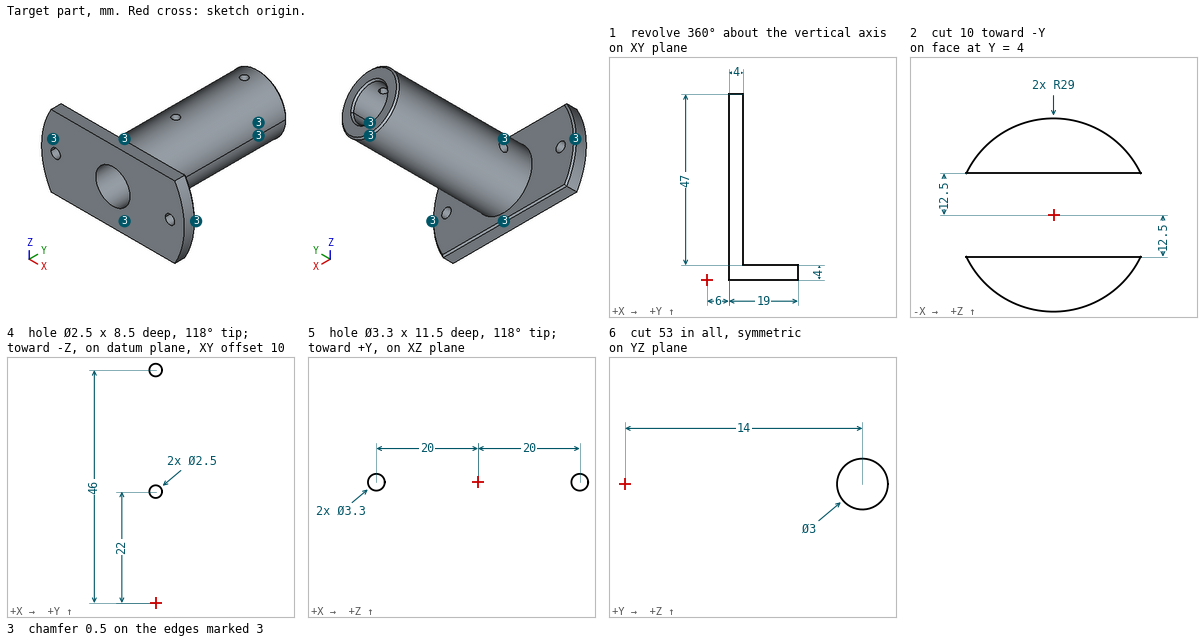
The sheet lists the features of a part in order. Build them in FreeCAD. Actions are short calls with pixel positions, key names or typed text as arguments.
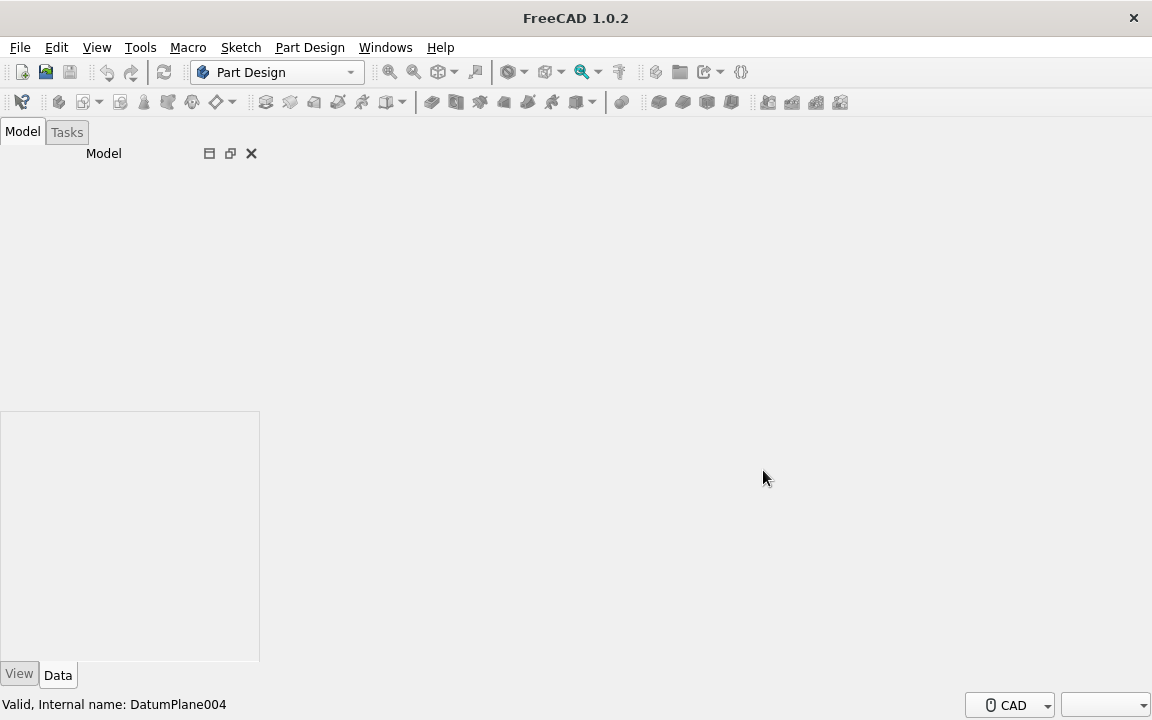
click(22, 72)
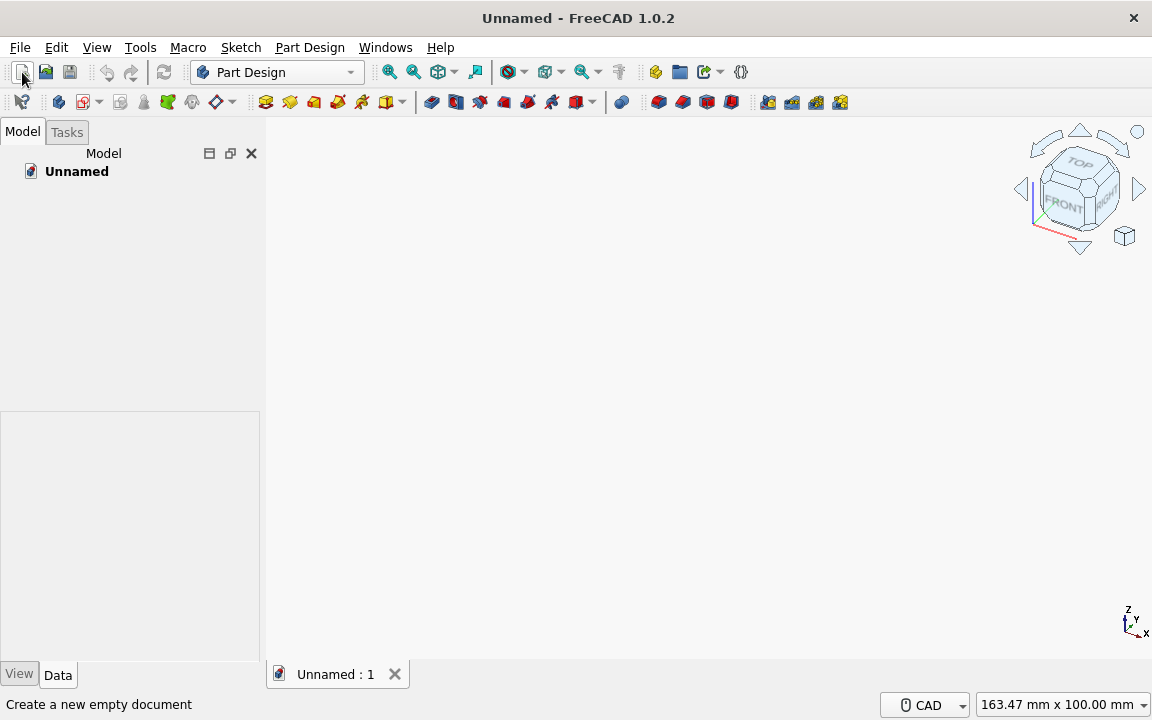
click(84, 102)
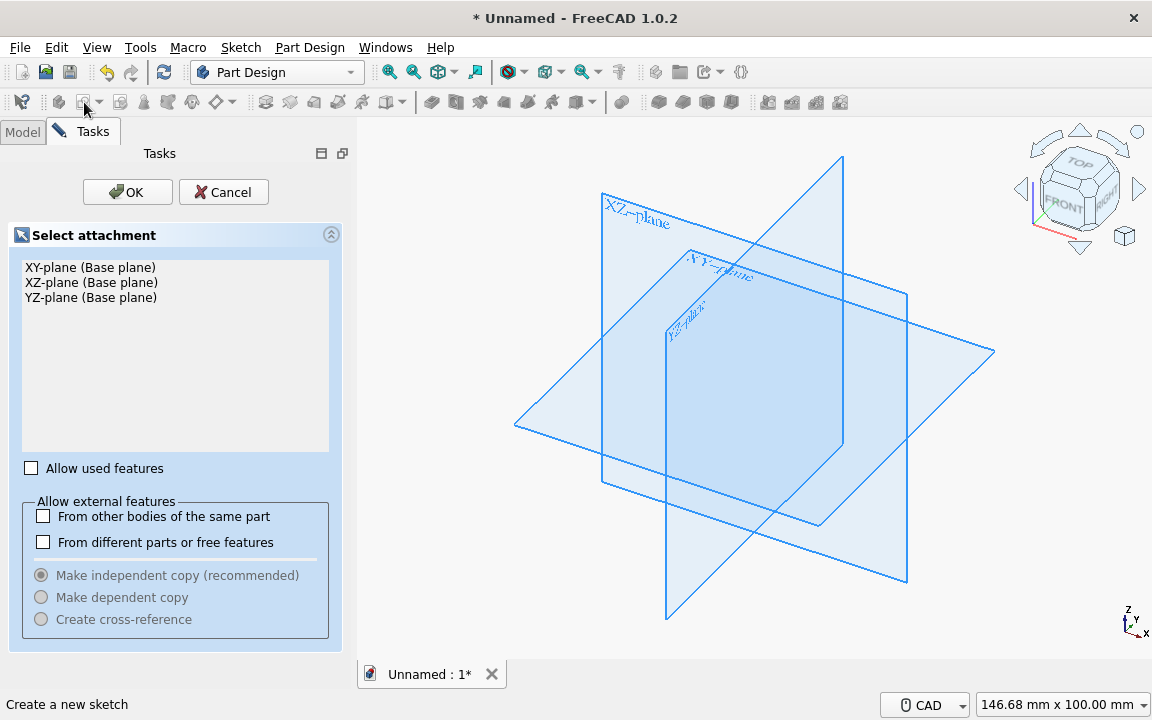
click(82, 268)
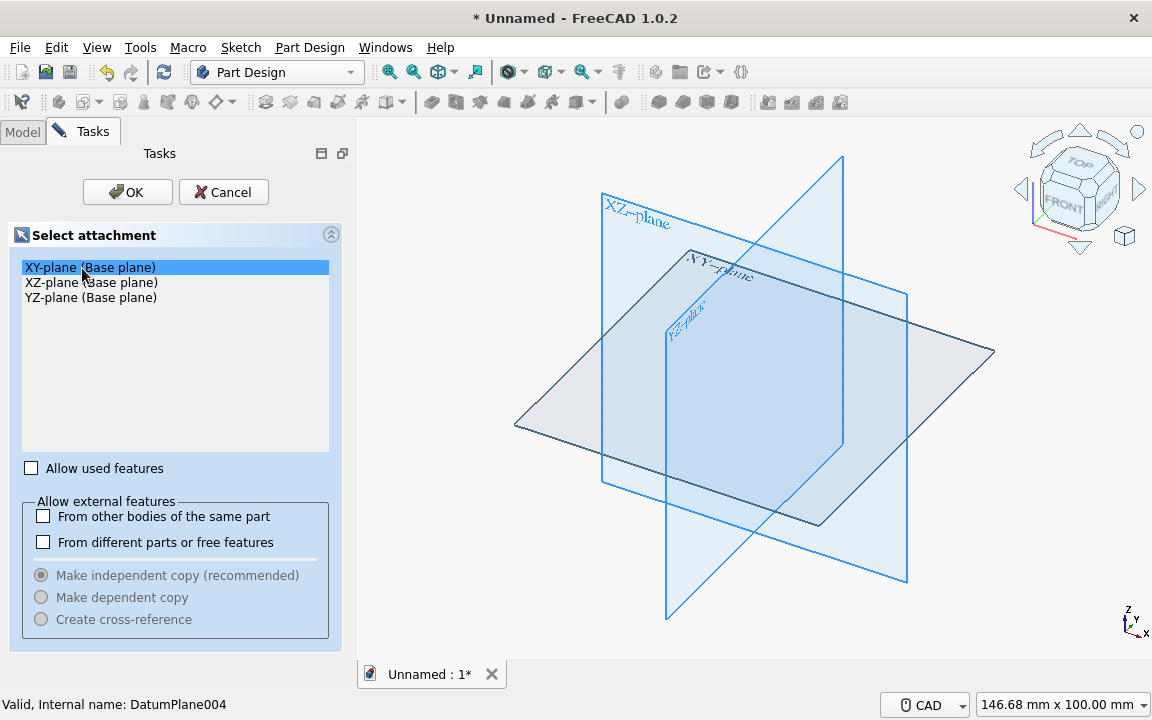
click(128, 192)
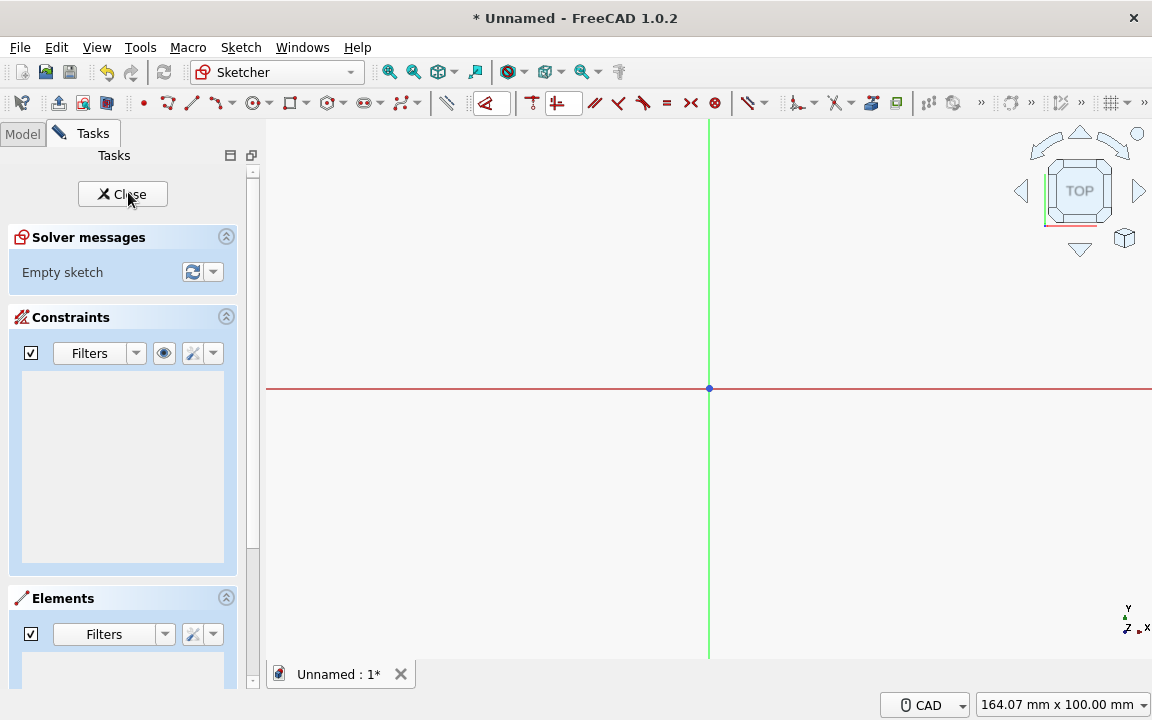
scroll(294, 631, down, 1)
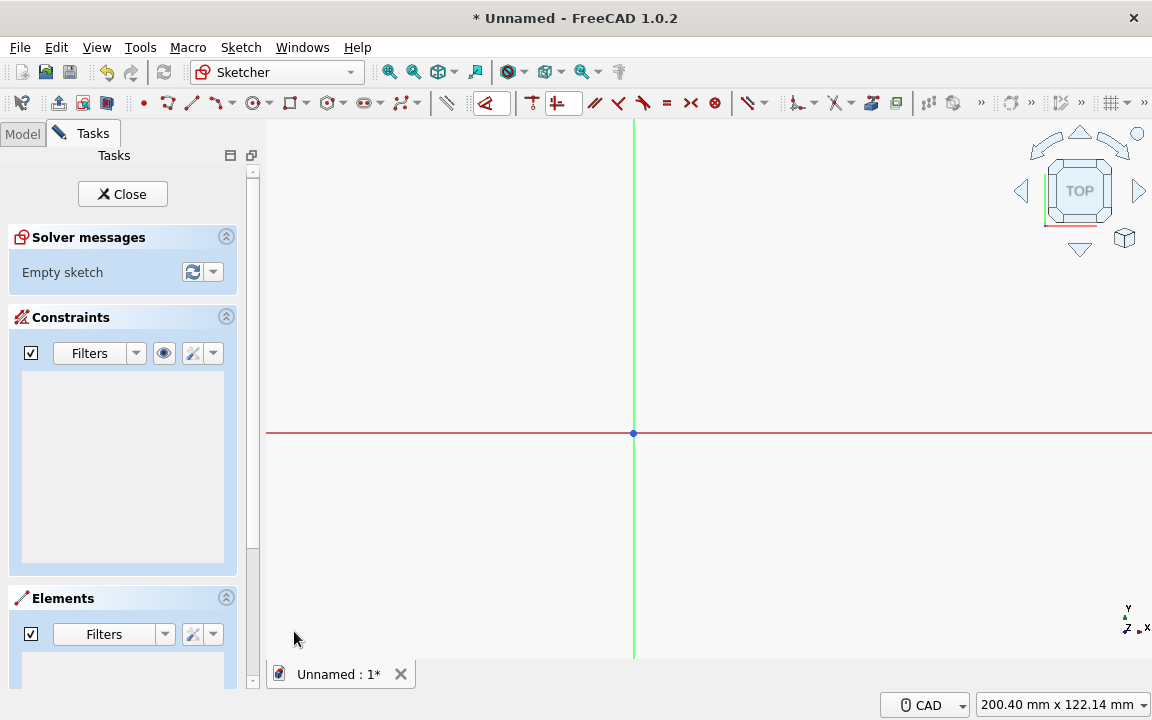
scroll(788, 181, up, 2)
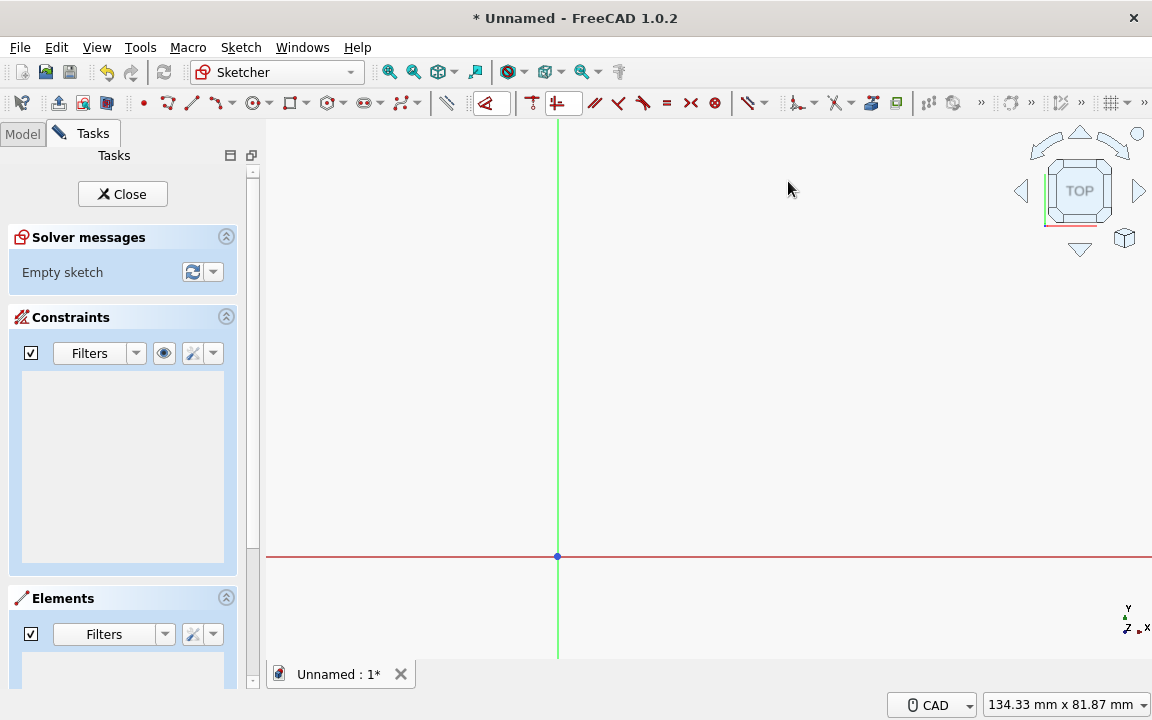
click(168, 104)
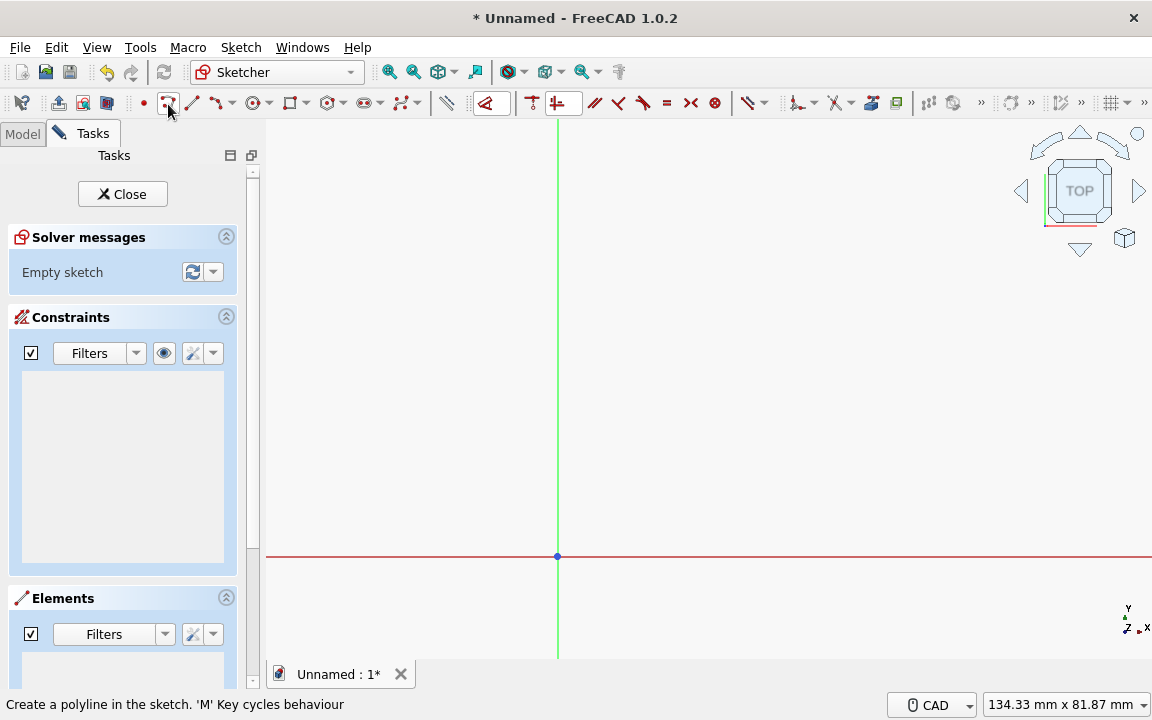
click(597, 557)
click(723, 548)
click(723, 531)
click(624, 531)
click(624, 221)
click(597, 221)
click(597, 557)
key(Escape)
key(Escape)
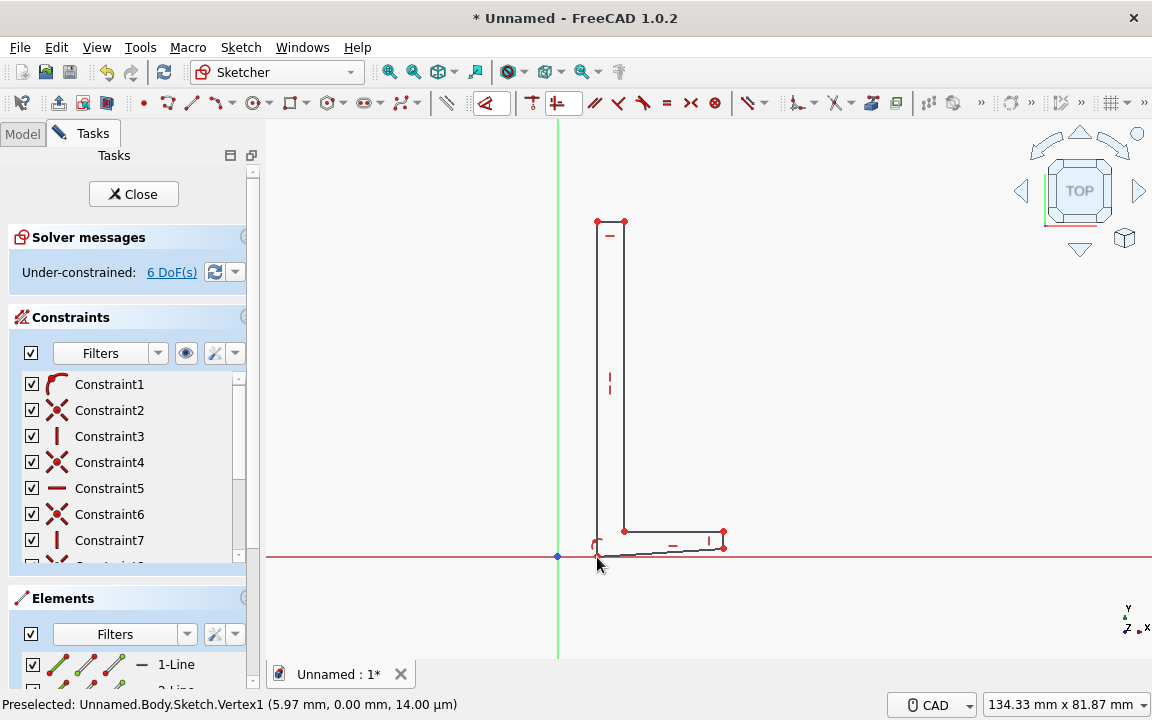
click(635, 555)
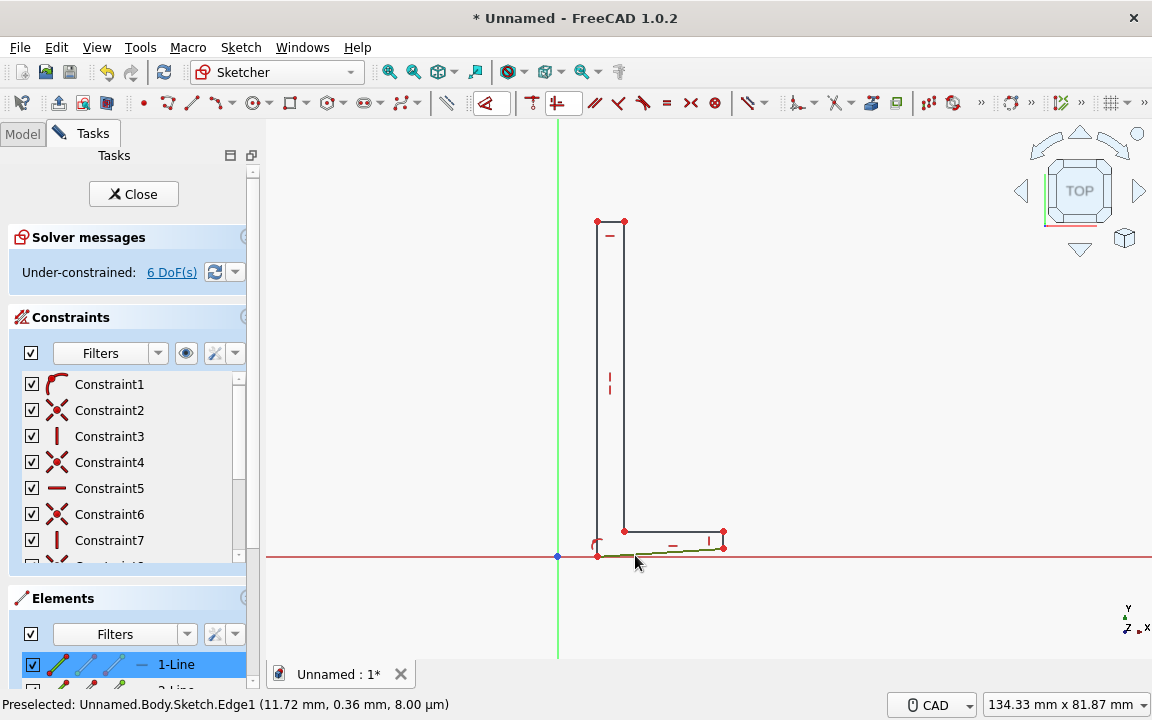
key(h)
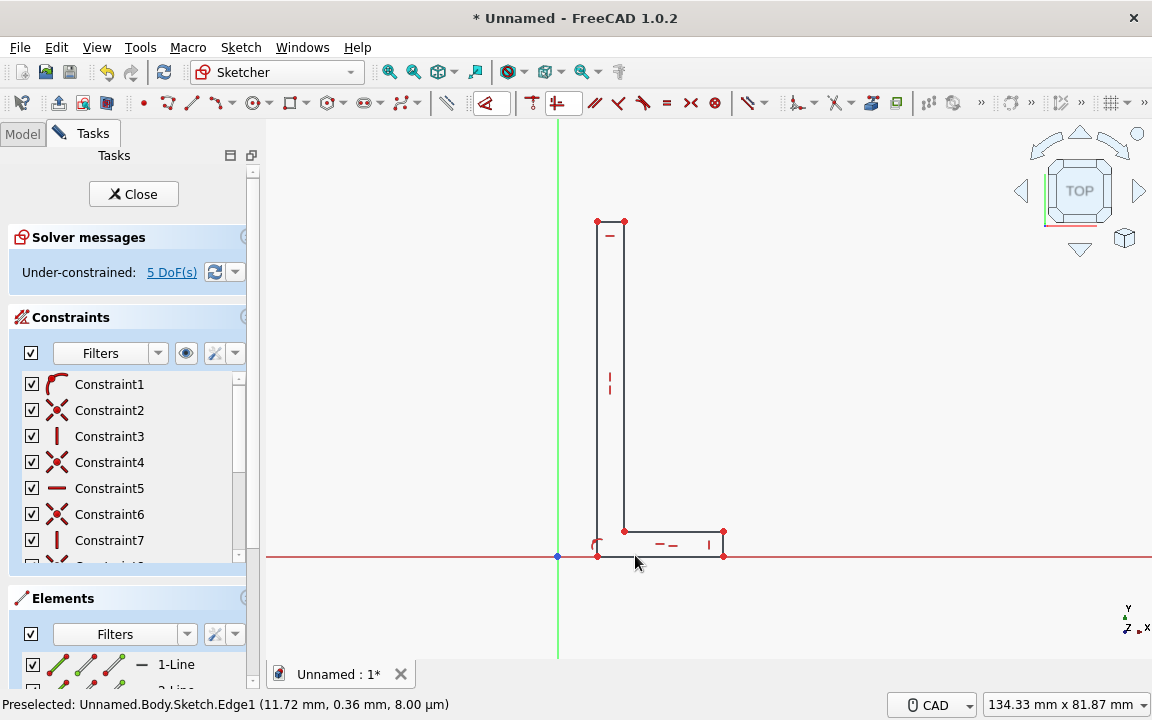
click(486, 104)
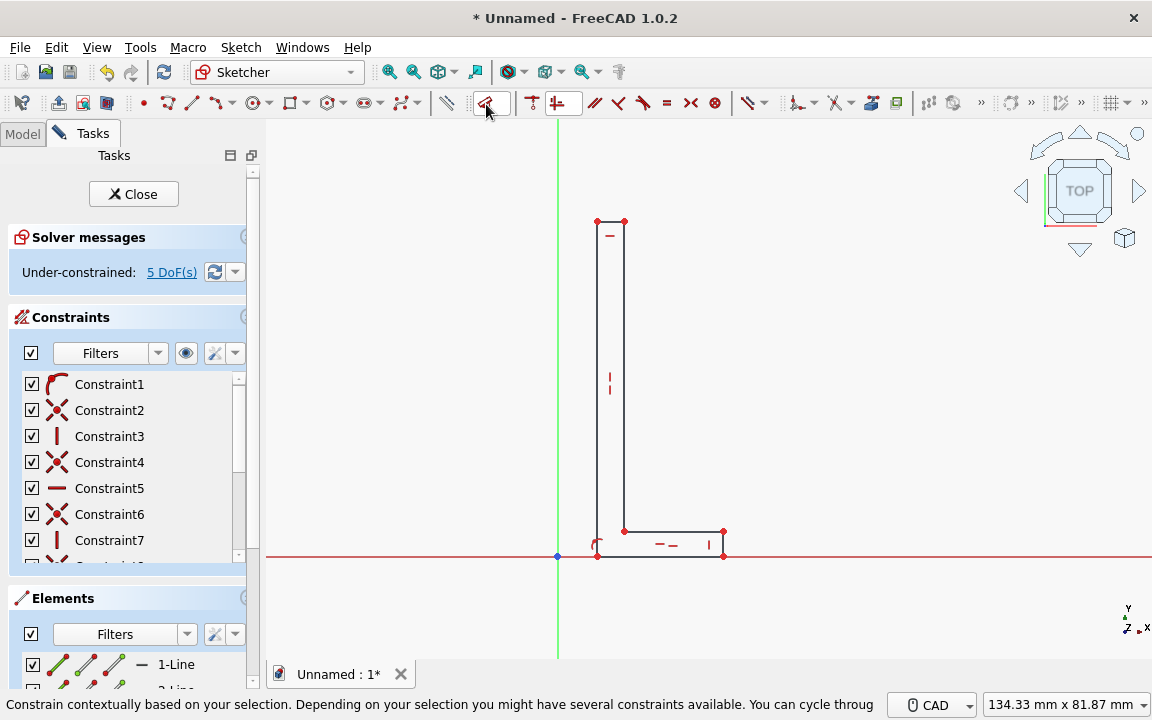
scroll(723, 547, up, 3)